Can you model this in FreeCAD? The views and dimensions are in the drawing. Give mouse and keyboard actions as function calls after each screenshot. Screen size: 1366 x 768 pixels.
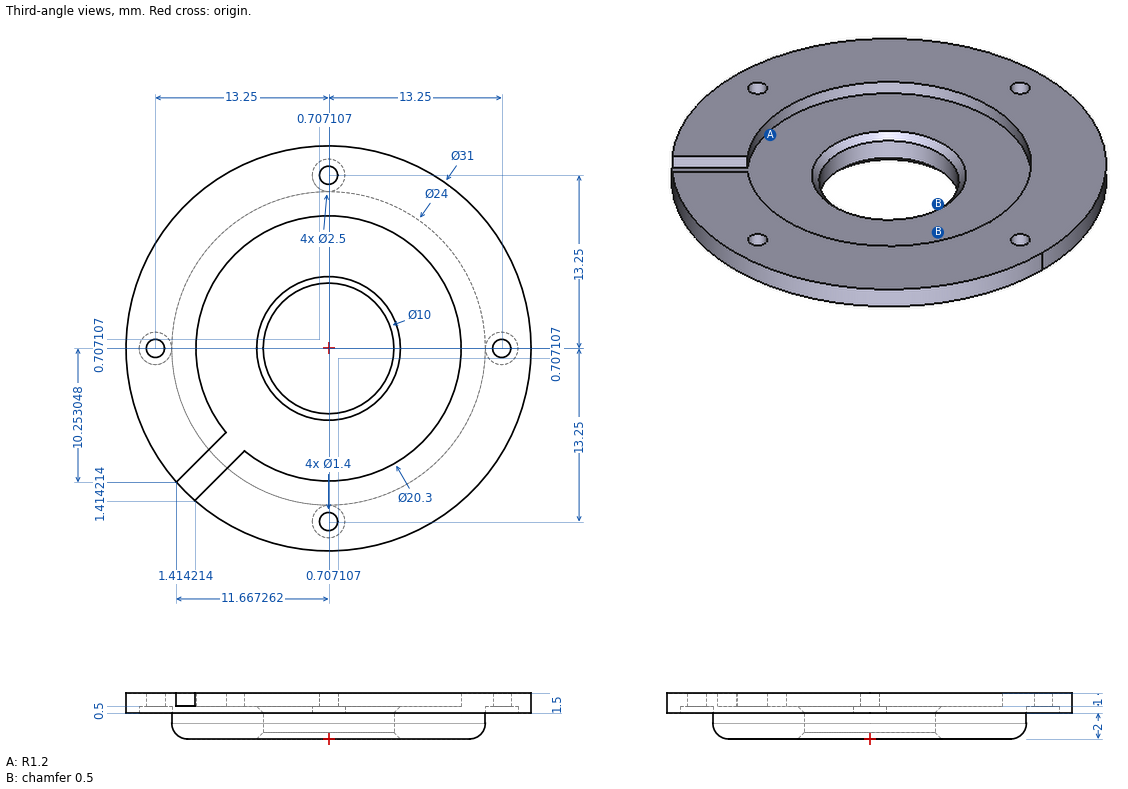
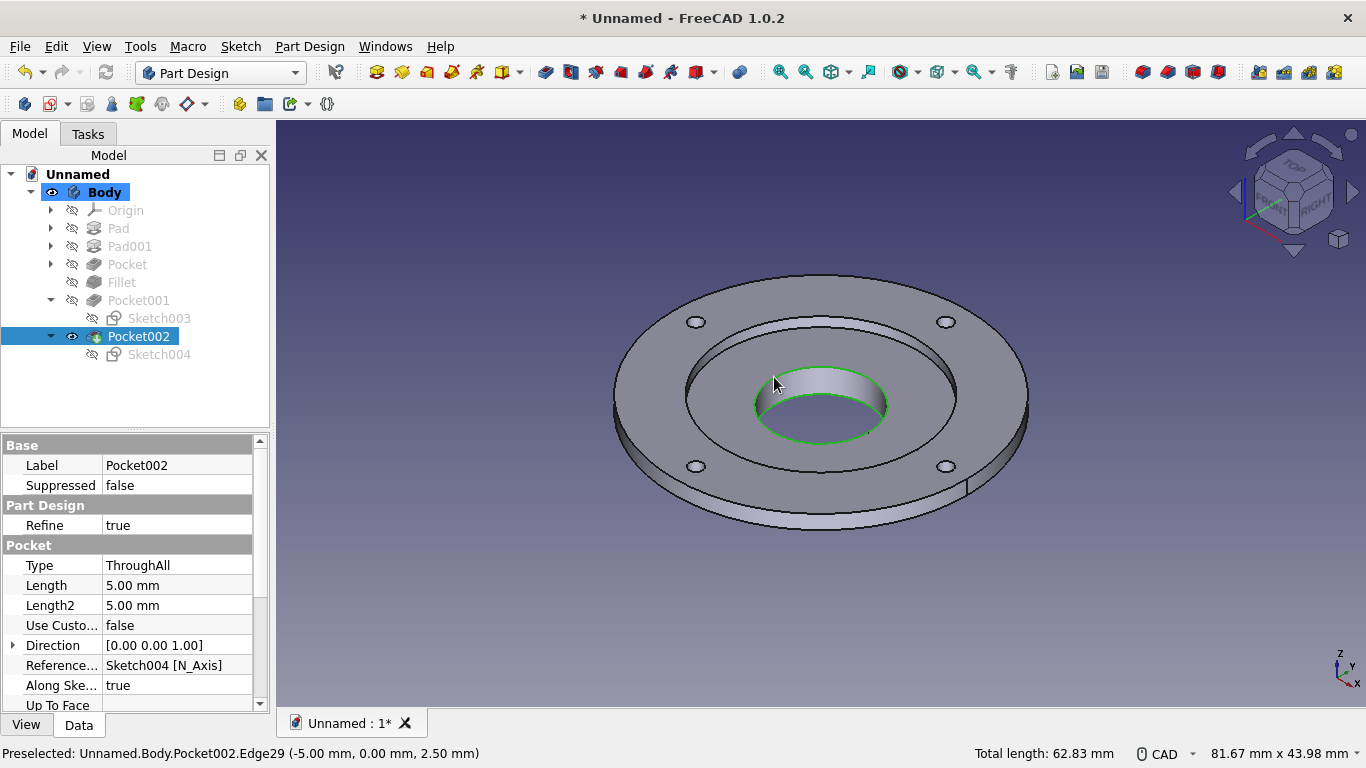
click(1168, 72)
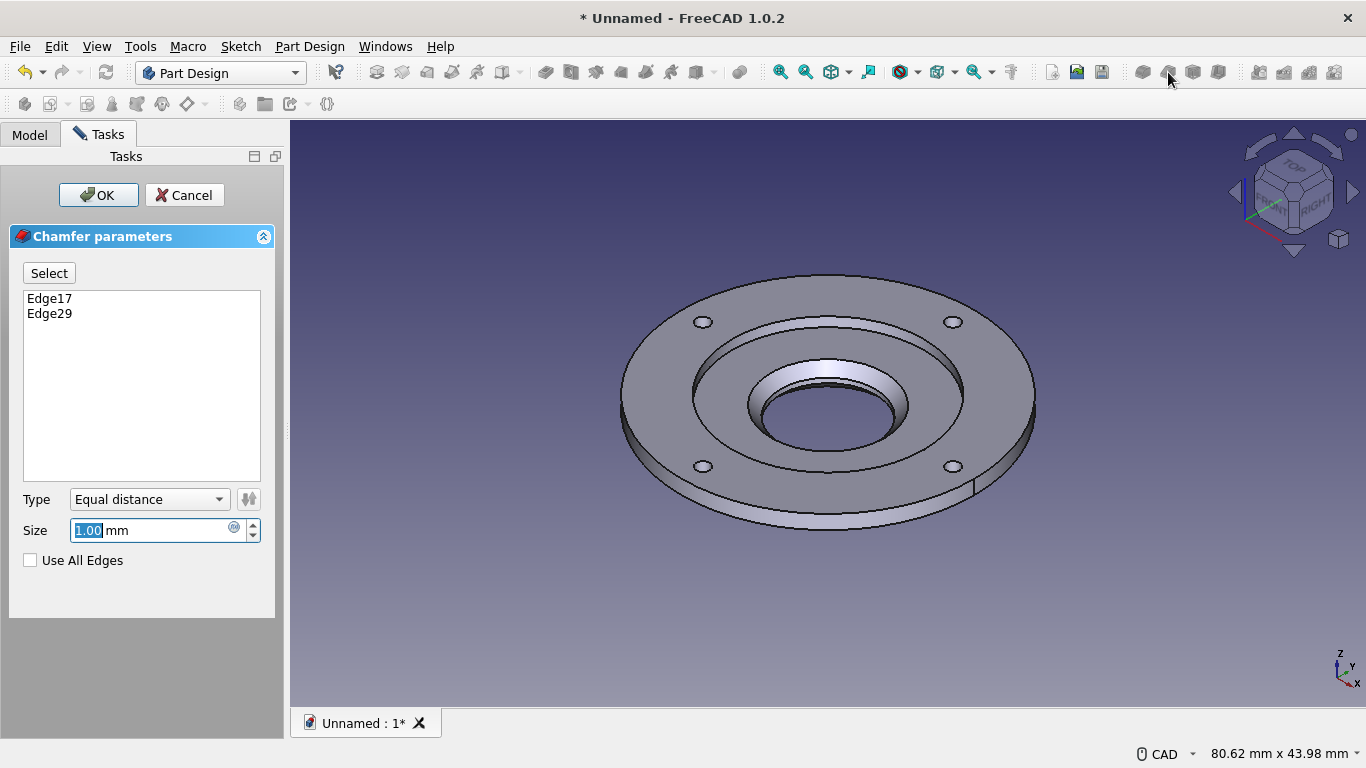
text(0.5)
key(Tab)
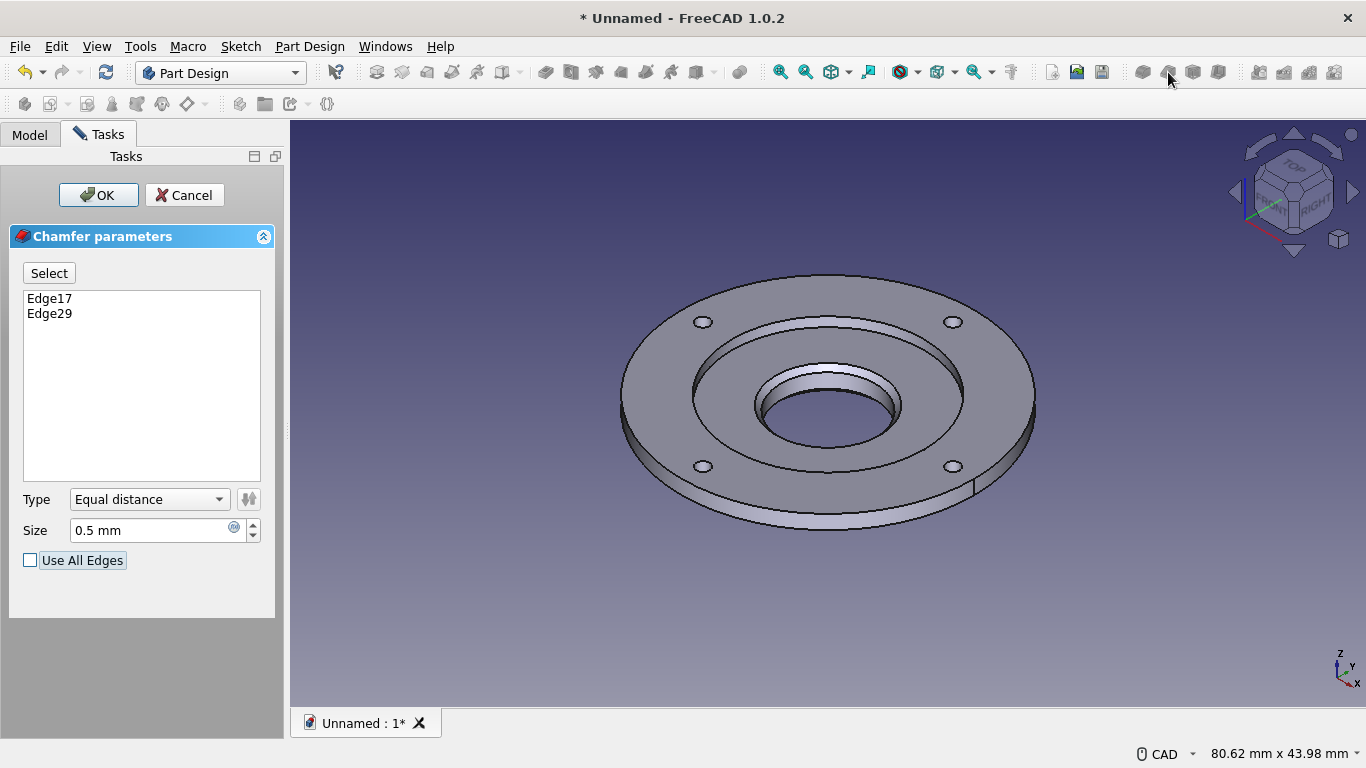
click(99, 195)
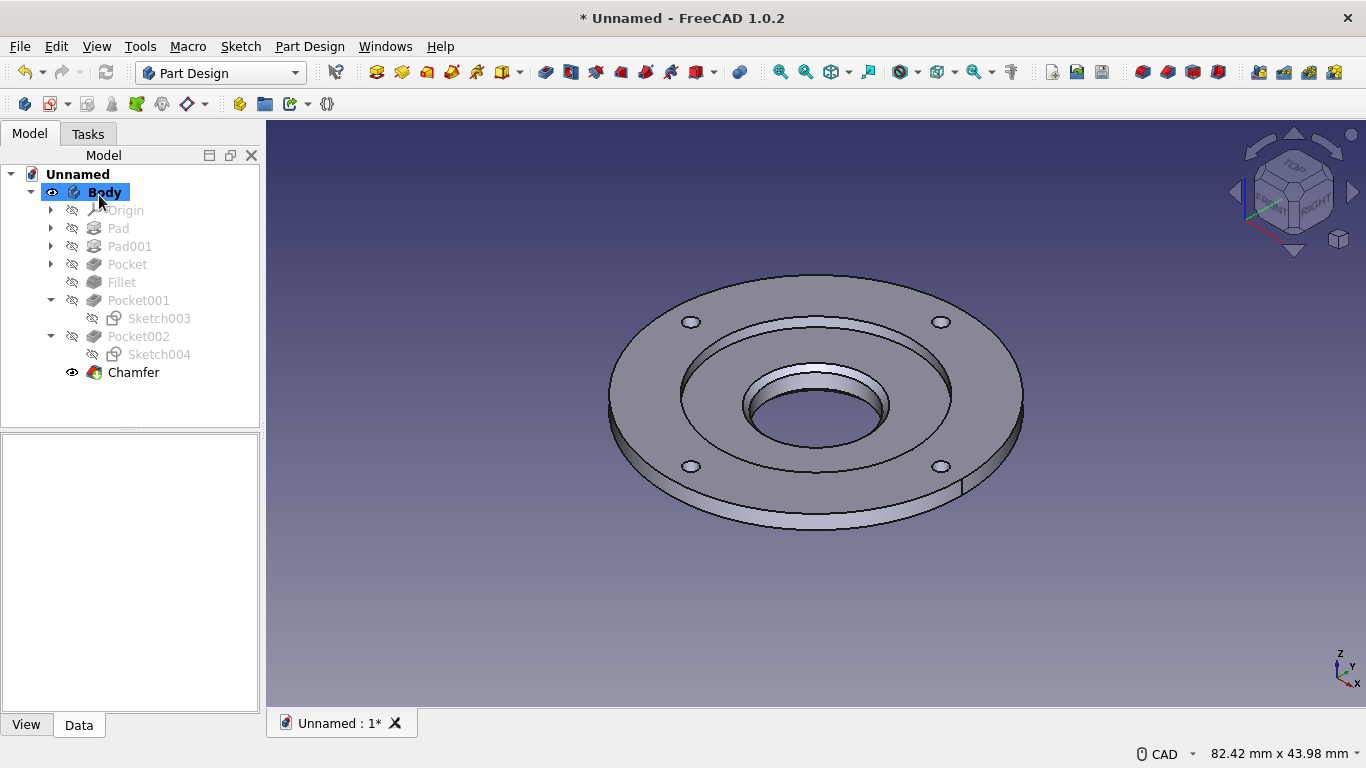
click(816, 490)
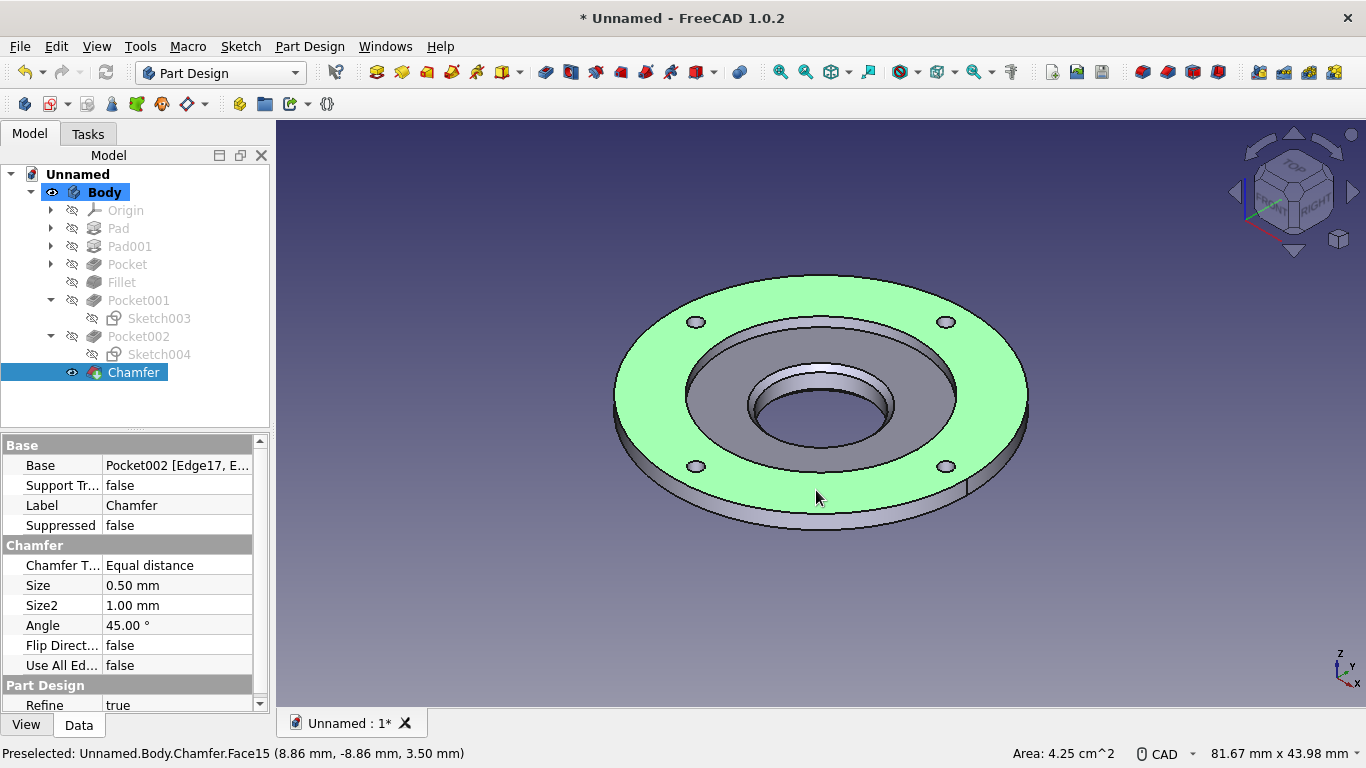
click(50, 104)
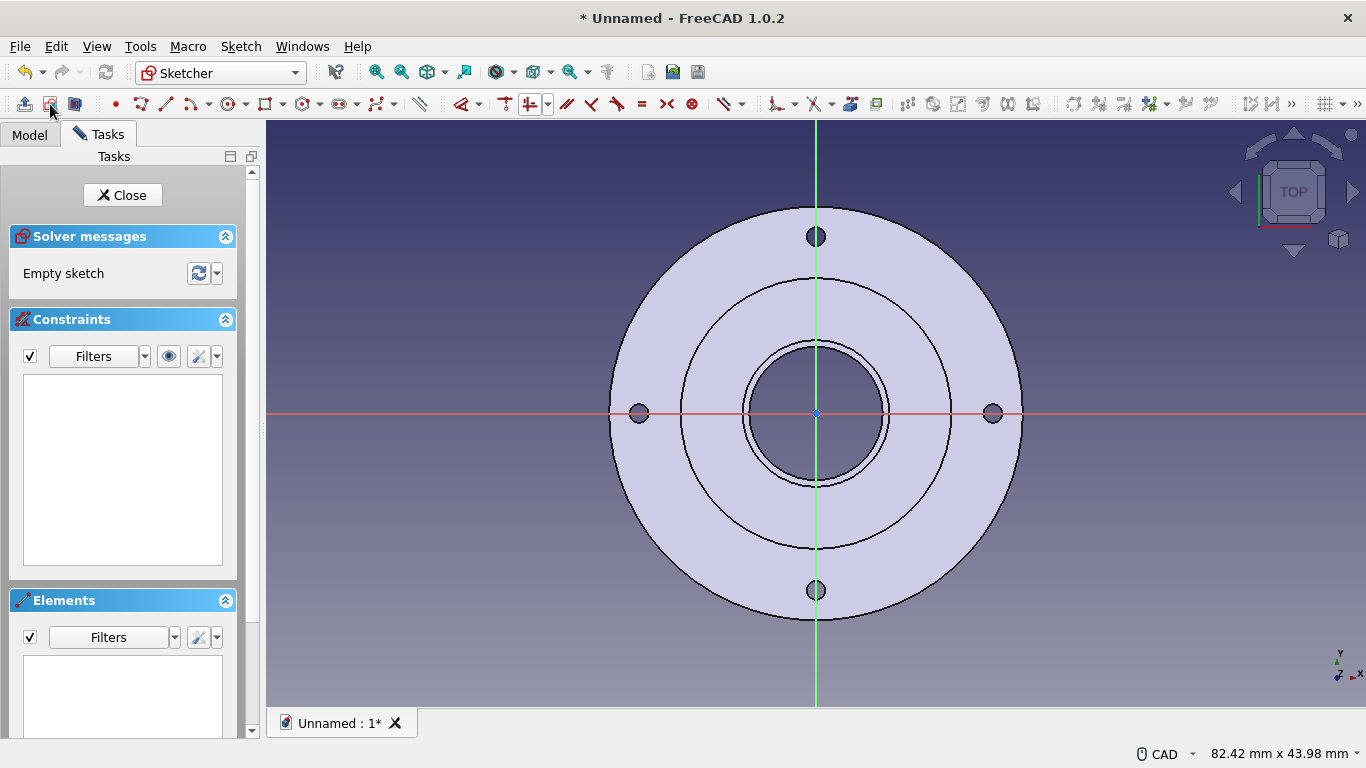
scroll(739, 546, up, 4)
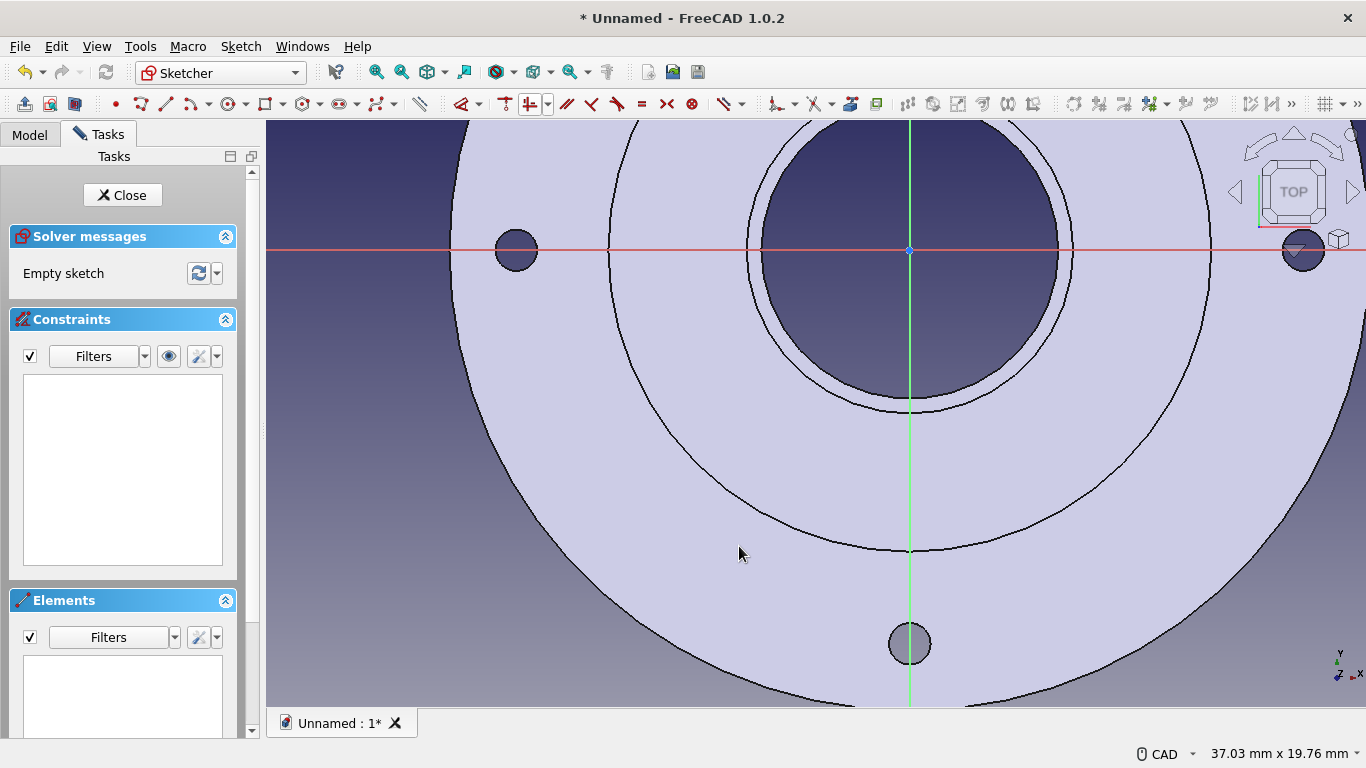
key(g)
key(m)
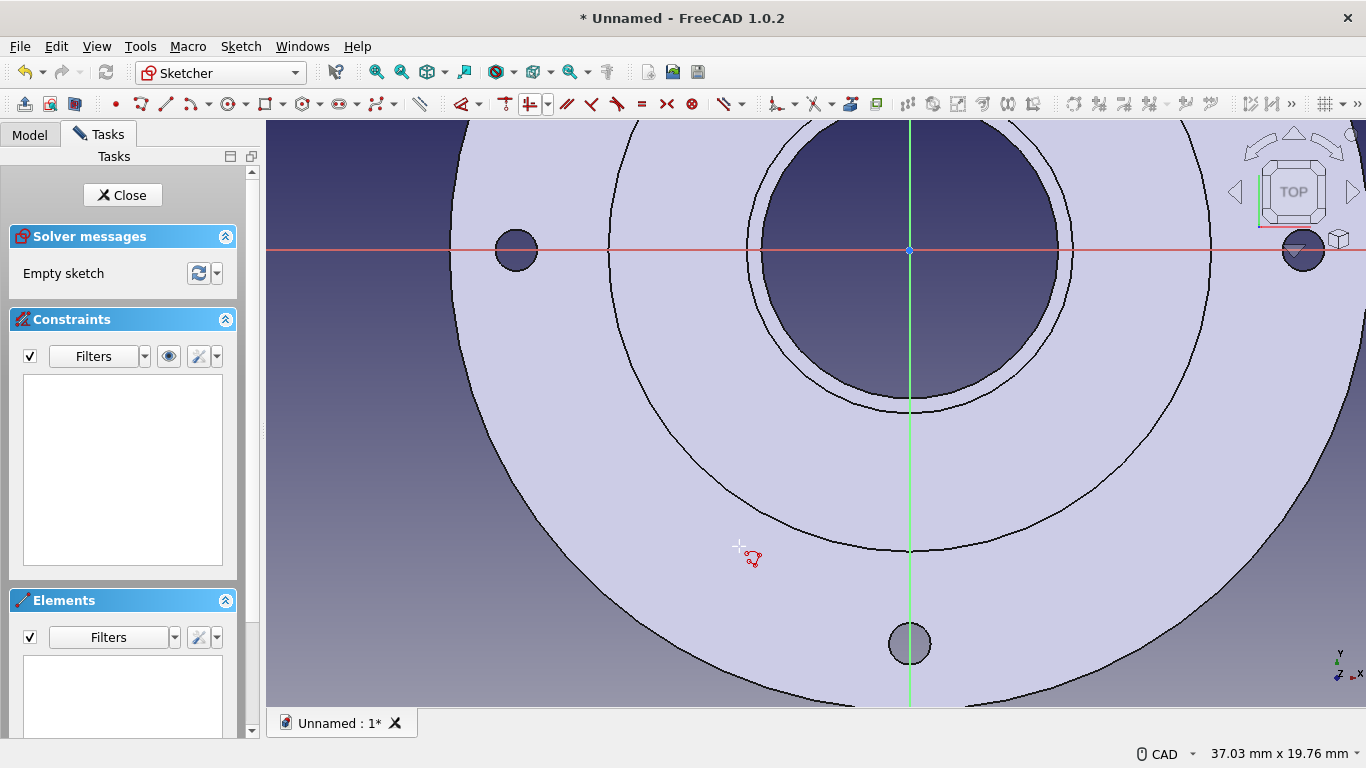
click(931, 271)
click(889, 229)
click(563, 555)
click(605, 597)
click(931, 272)
key(Escape)
key(Escape)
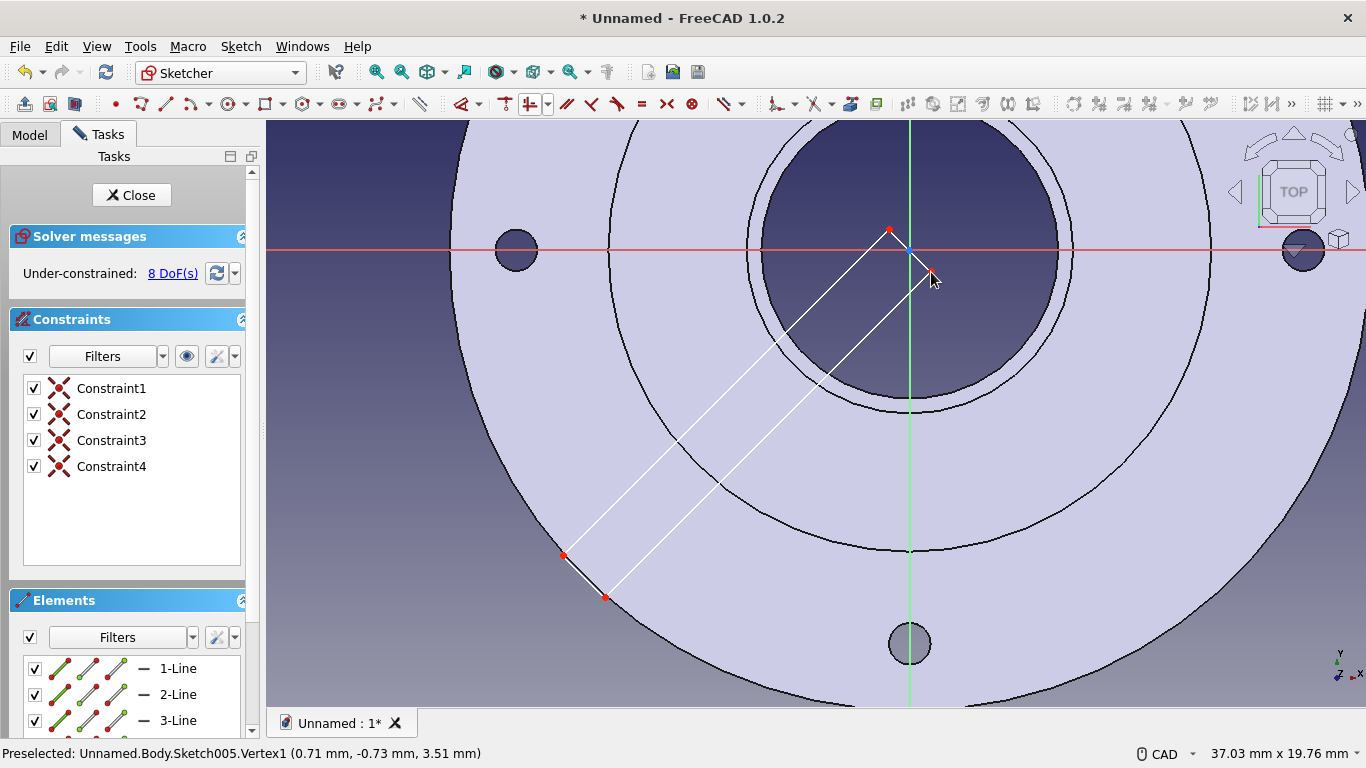
click(460, 104)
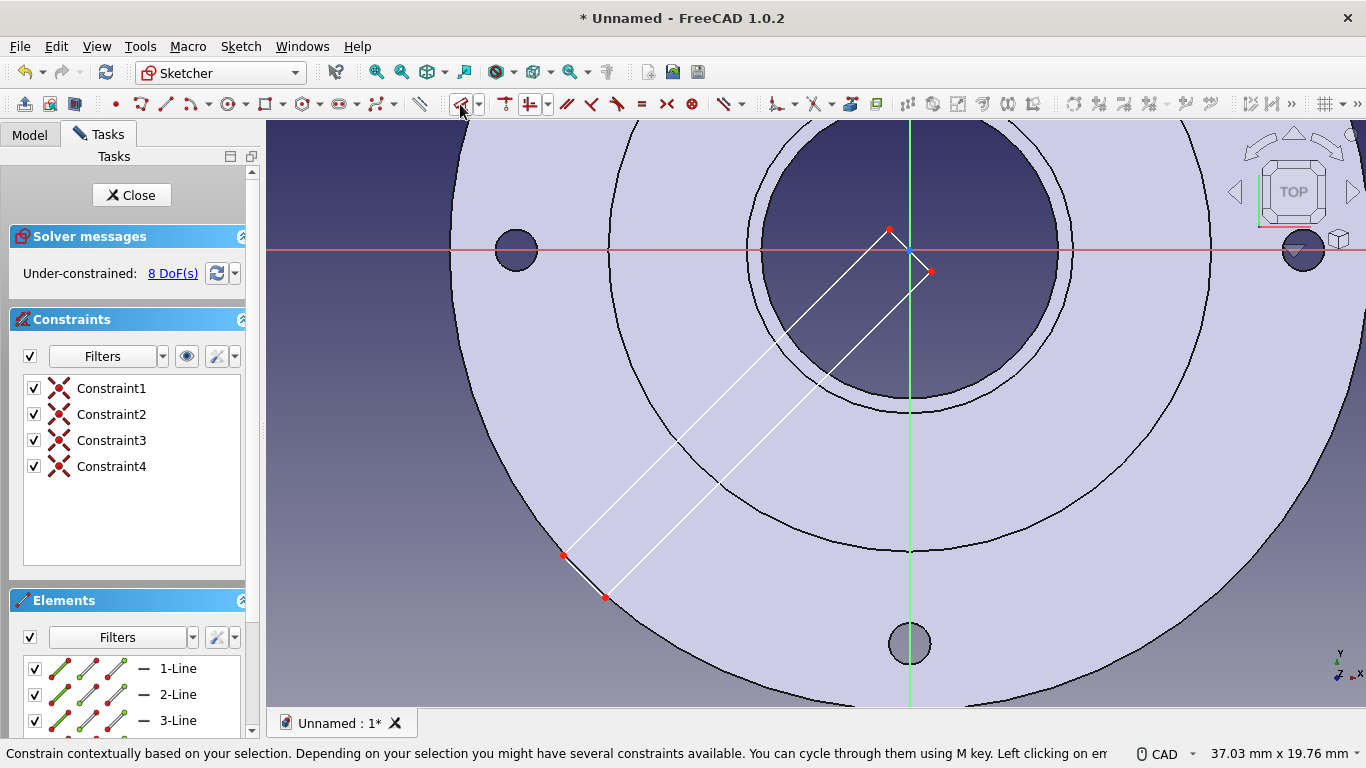
scroll(931, 272, up, 4)